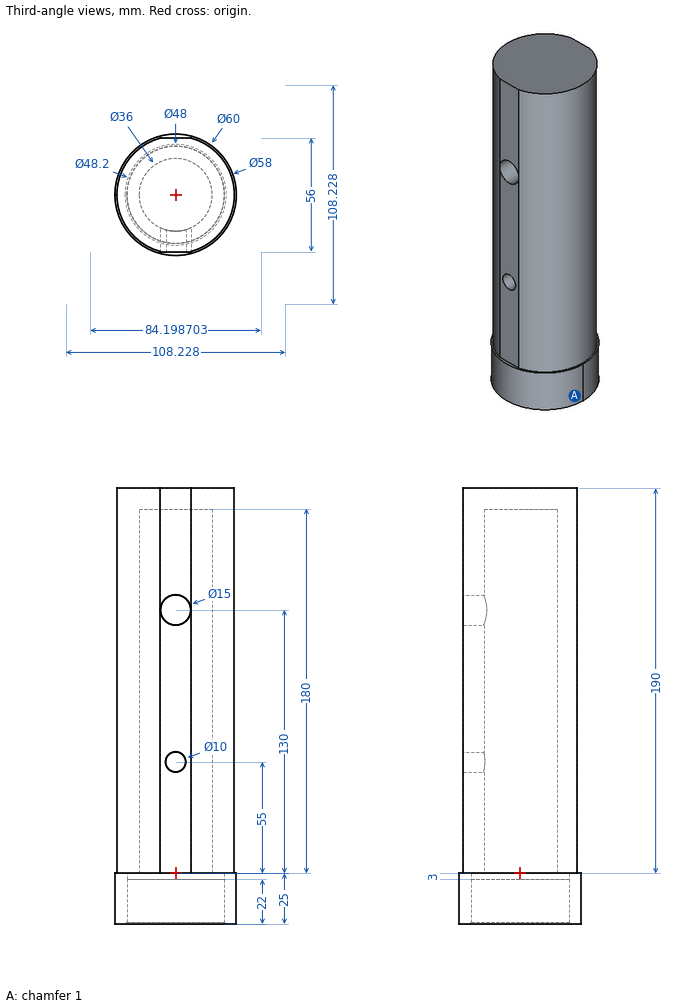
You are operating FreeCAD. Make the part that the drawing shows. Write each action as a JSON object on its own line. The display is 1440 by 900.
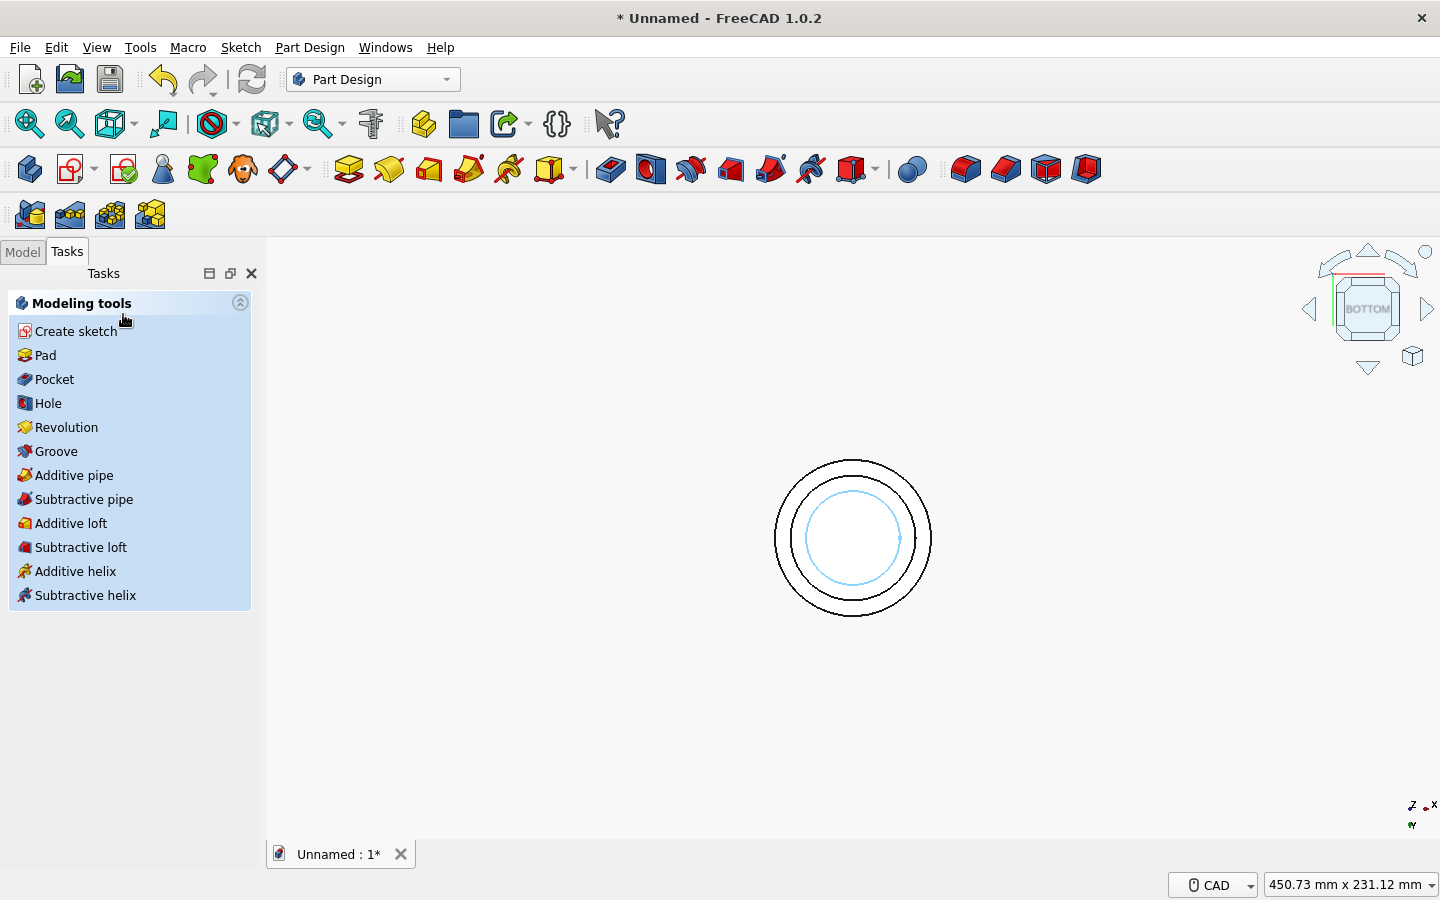
{"action": "left_click", "coordinate": [612, 170]}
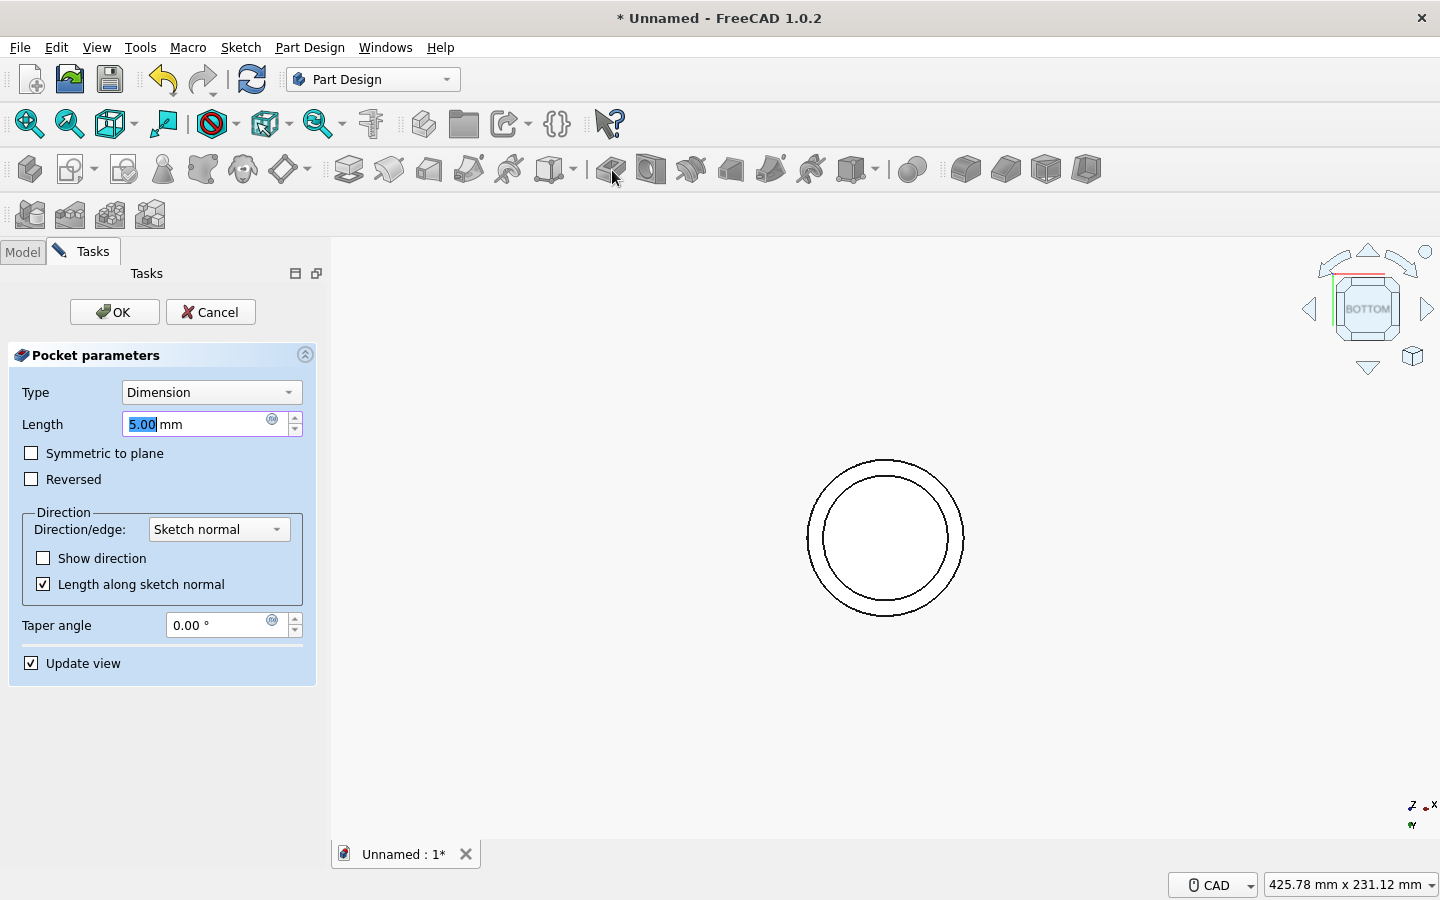
{"action": "type", "text": "180"}
{"action": "key", "text": "Tab"}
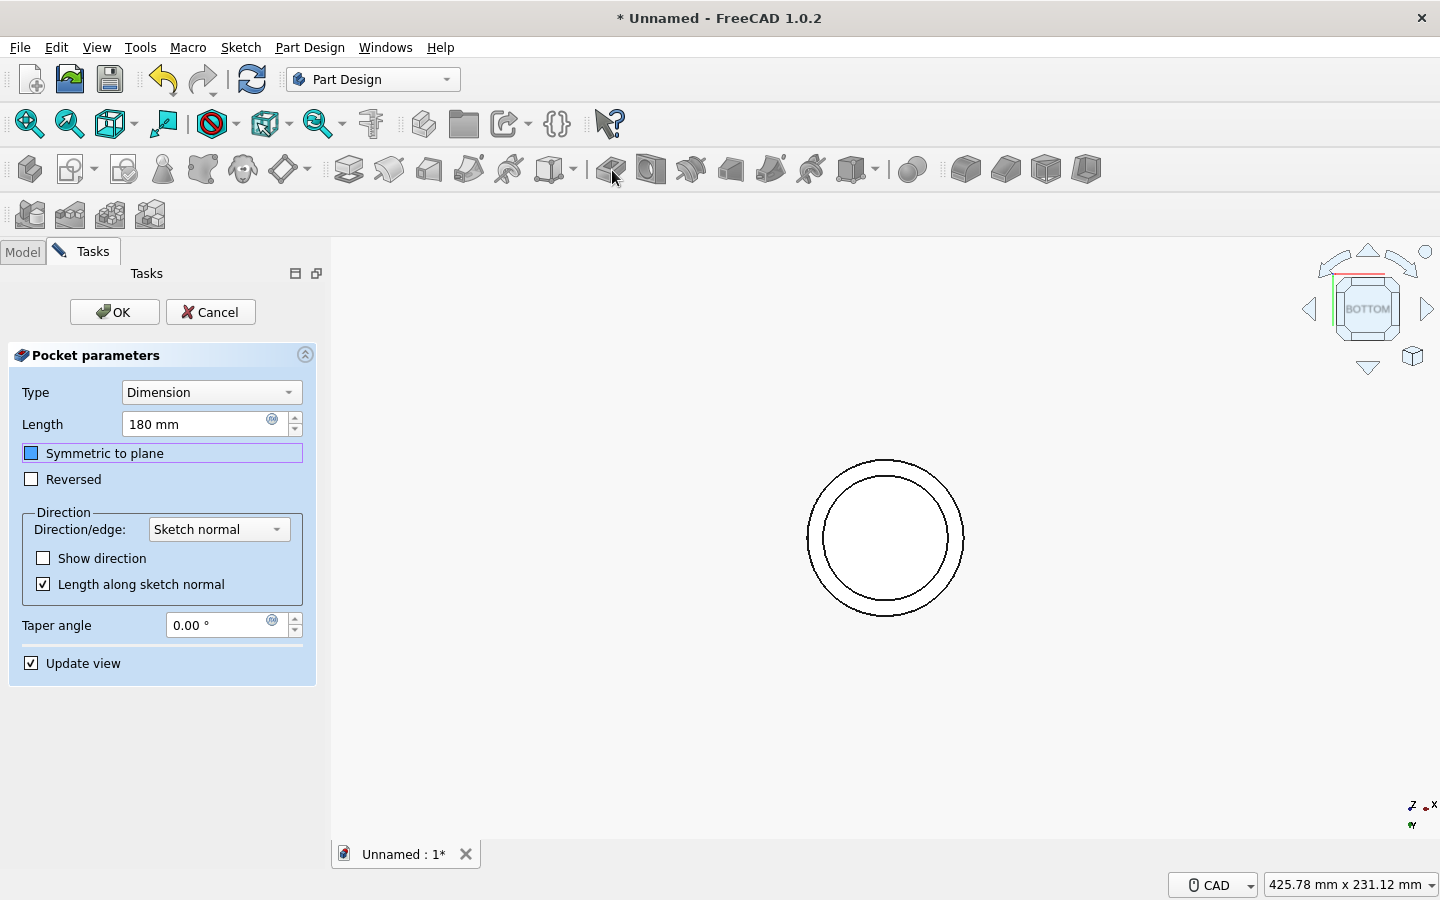
{"action": "left_click", "coordinate": [30, 479]}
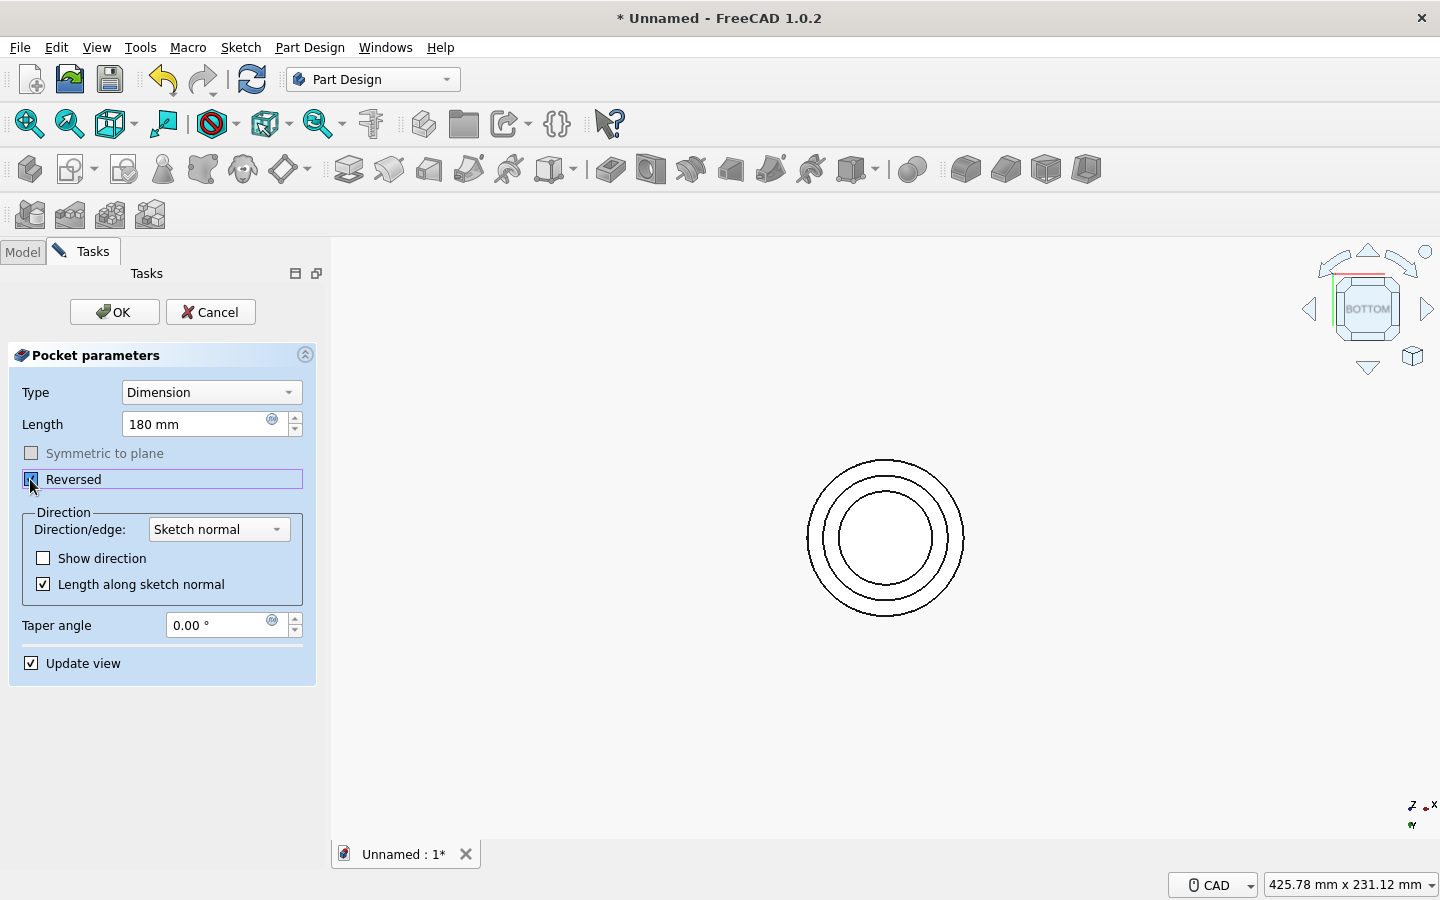
{"action": "left_click", "coordinate": [115, 312]}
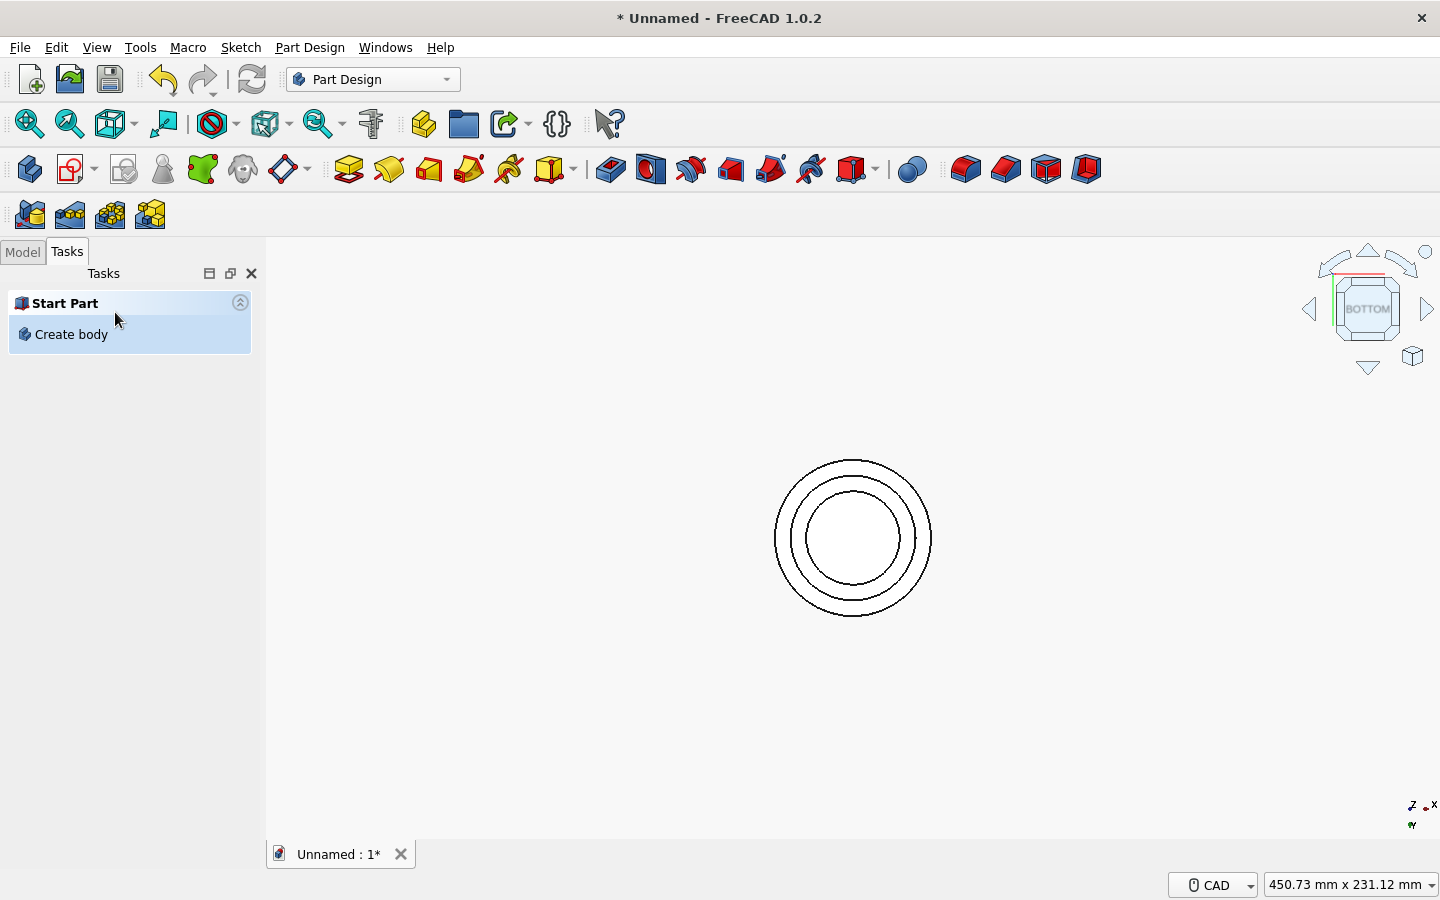
{"action": "left_click", "coordinate": [30, 124]}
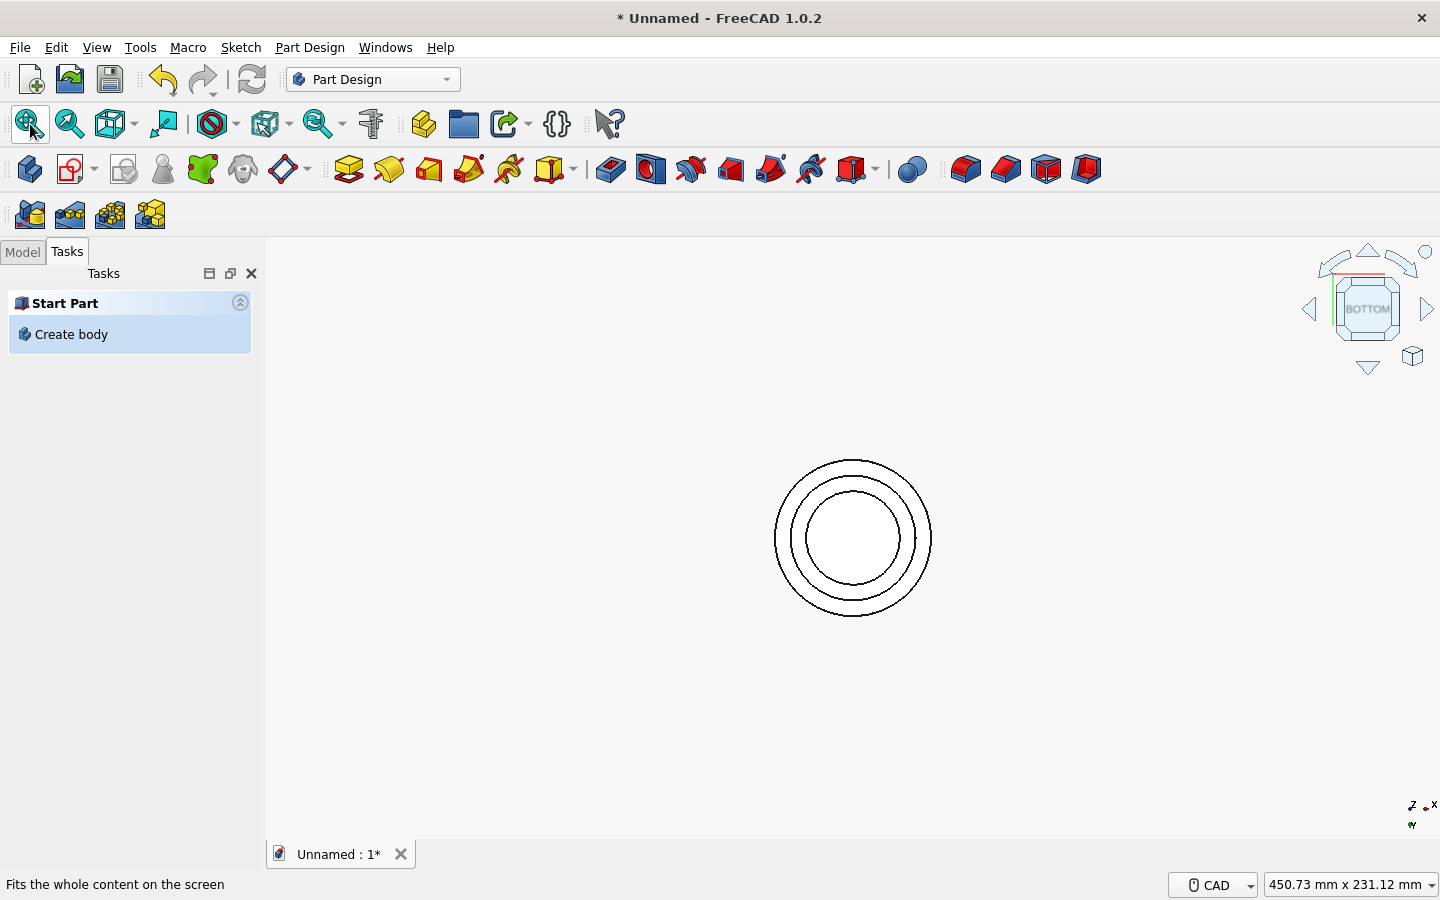
{"action": "left_click", "coordinate": [70, 170]}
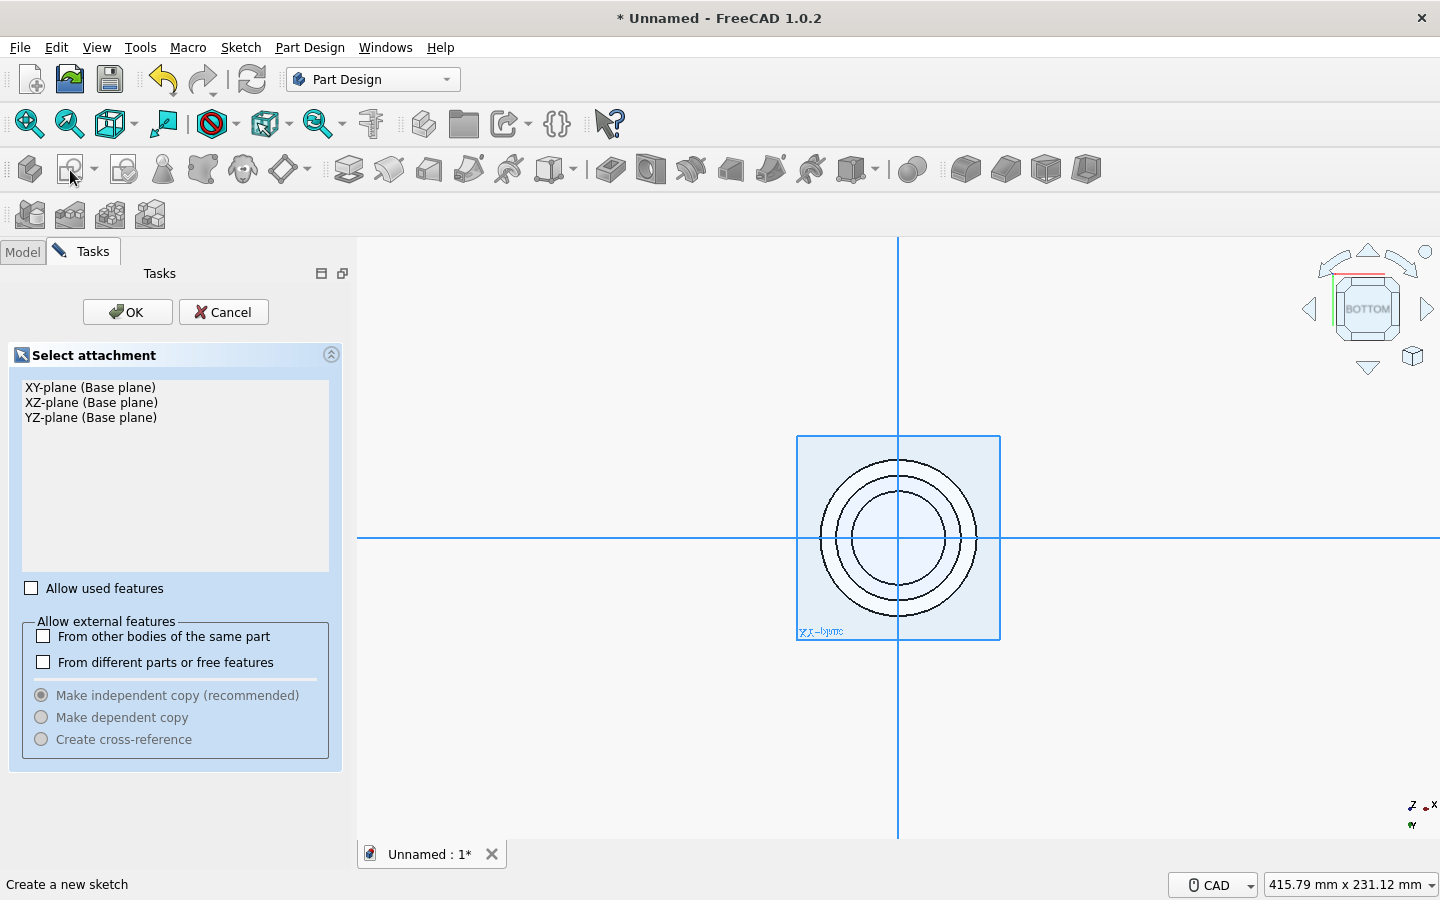
{"action": "left_click", "coordinate": [82, 402]}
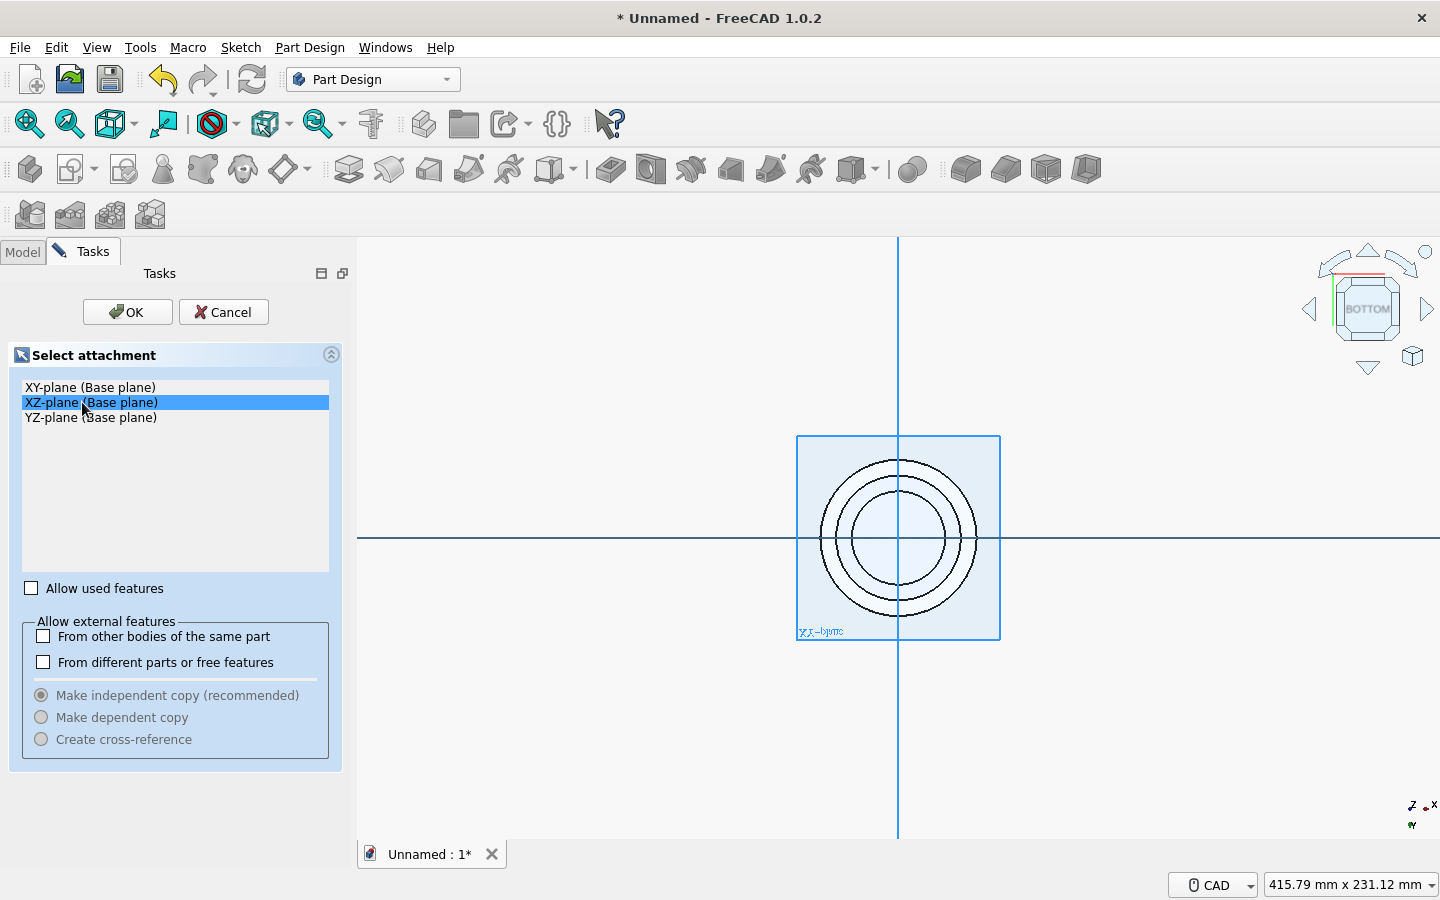
{"action": "left_click", "coordinate": [128, 312]}